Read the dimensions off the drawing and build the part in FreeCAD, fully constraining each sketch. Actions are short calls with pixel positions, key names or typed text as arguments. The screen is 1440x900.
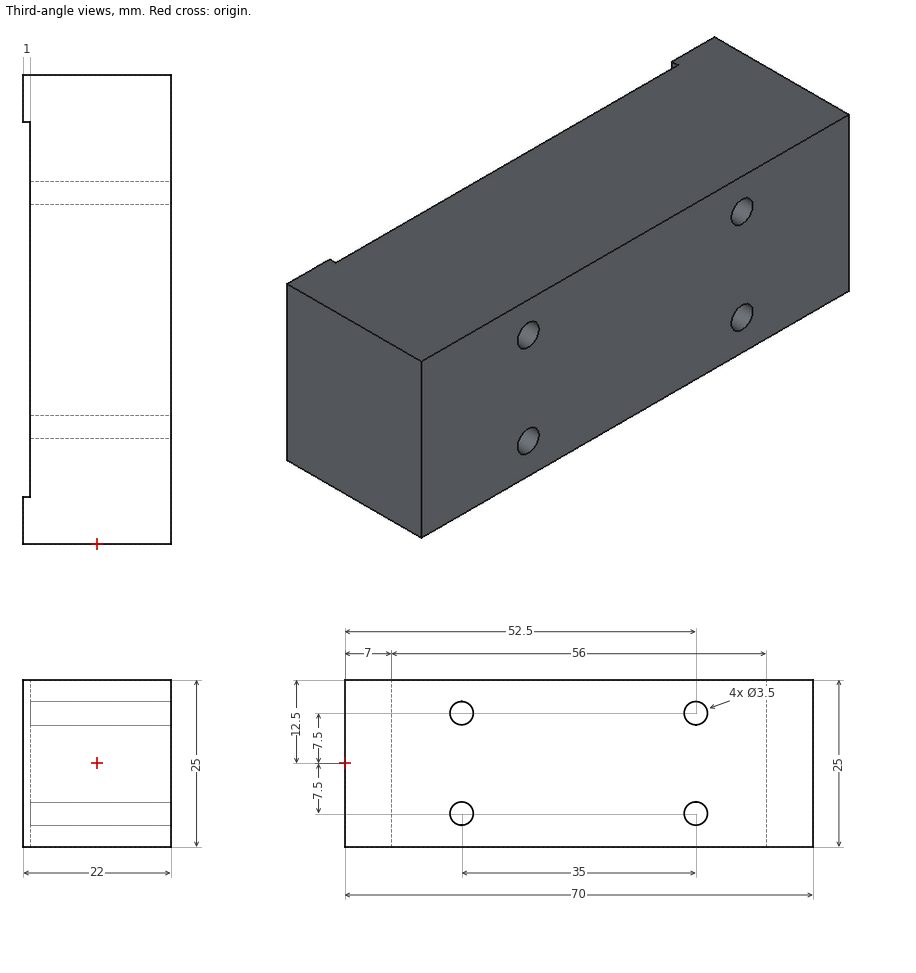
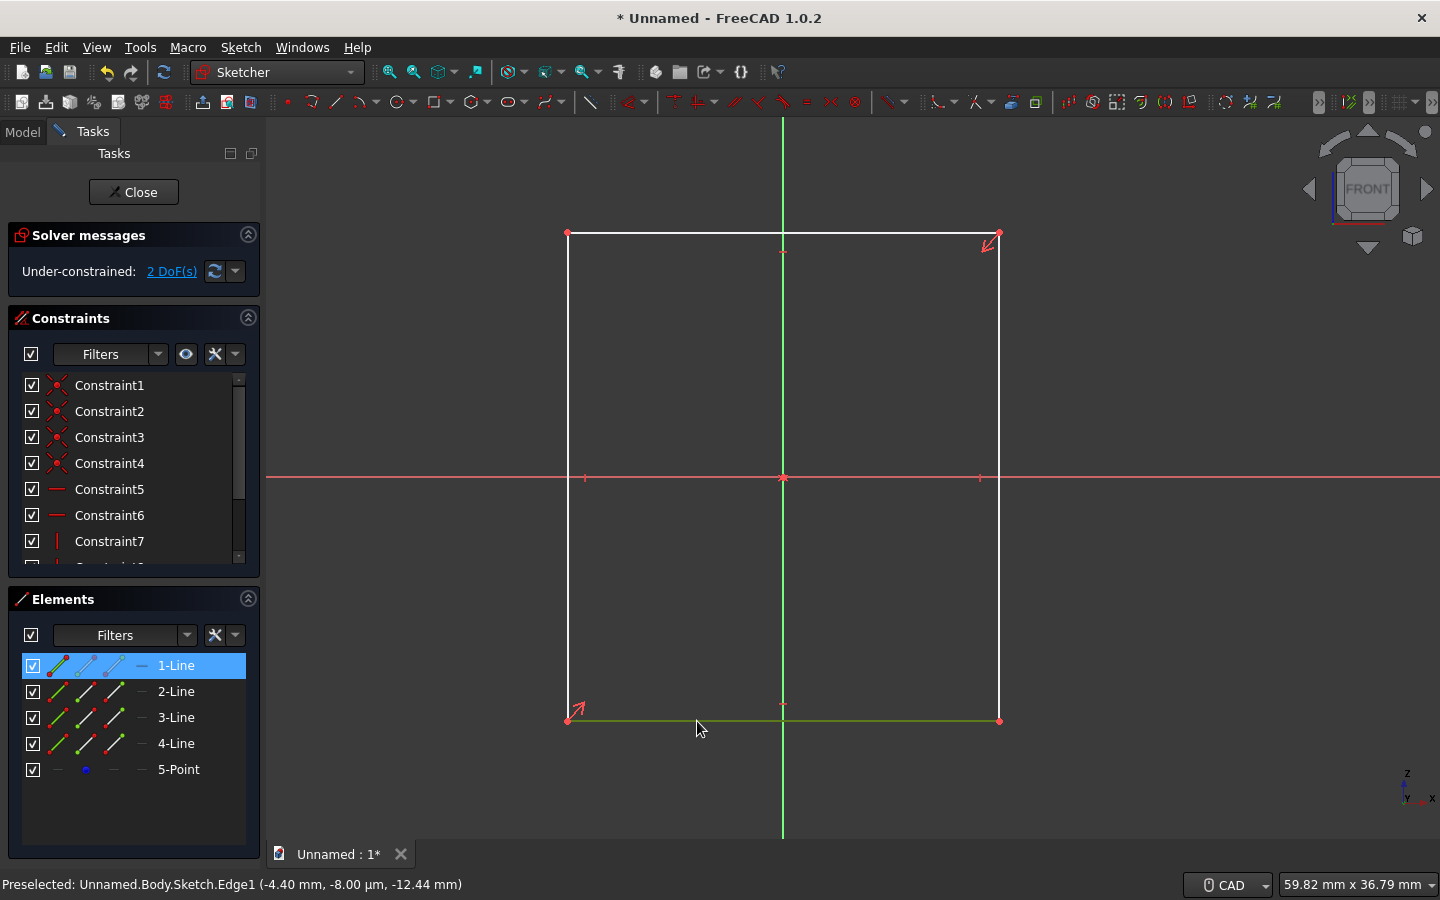
click(646, 102)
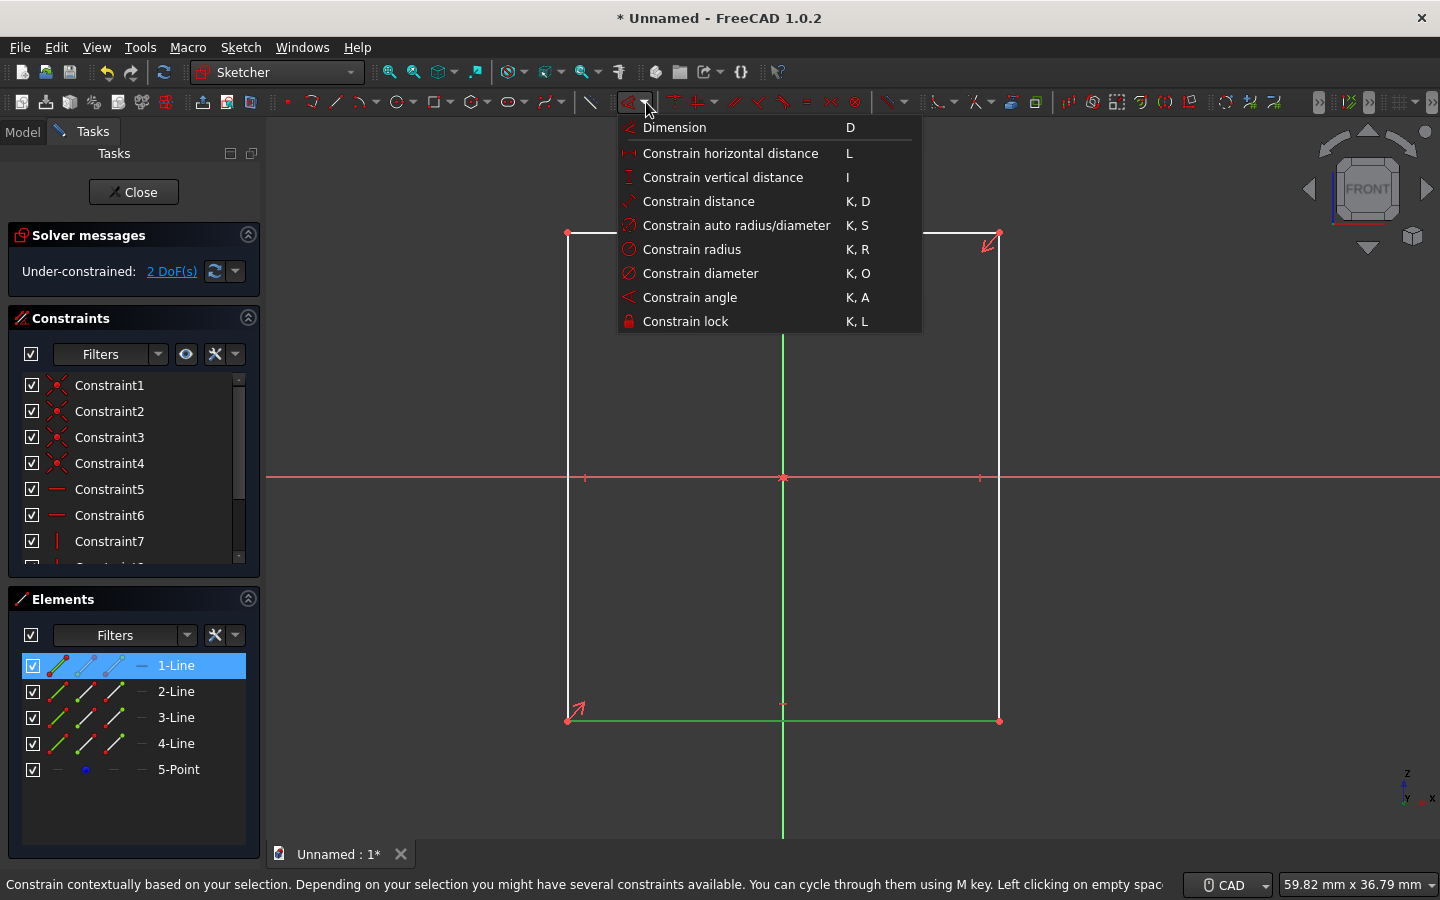
click(770, 153)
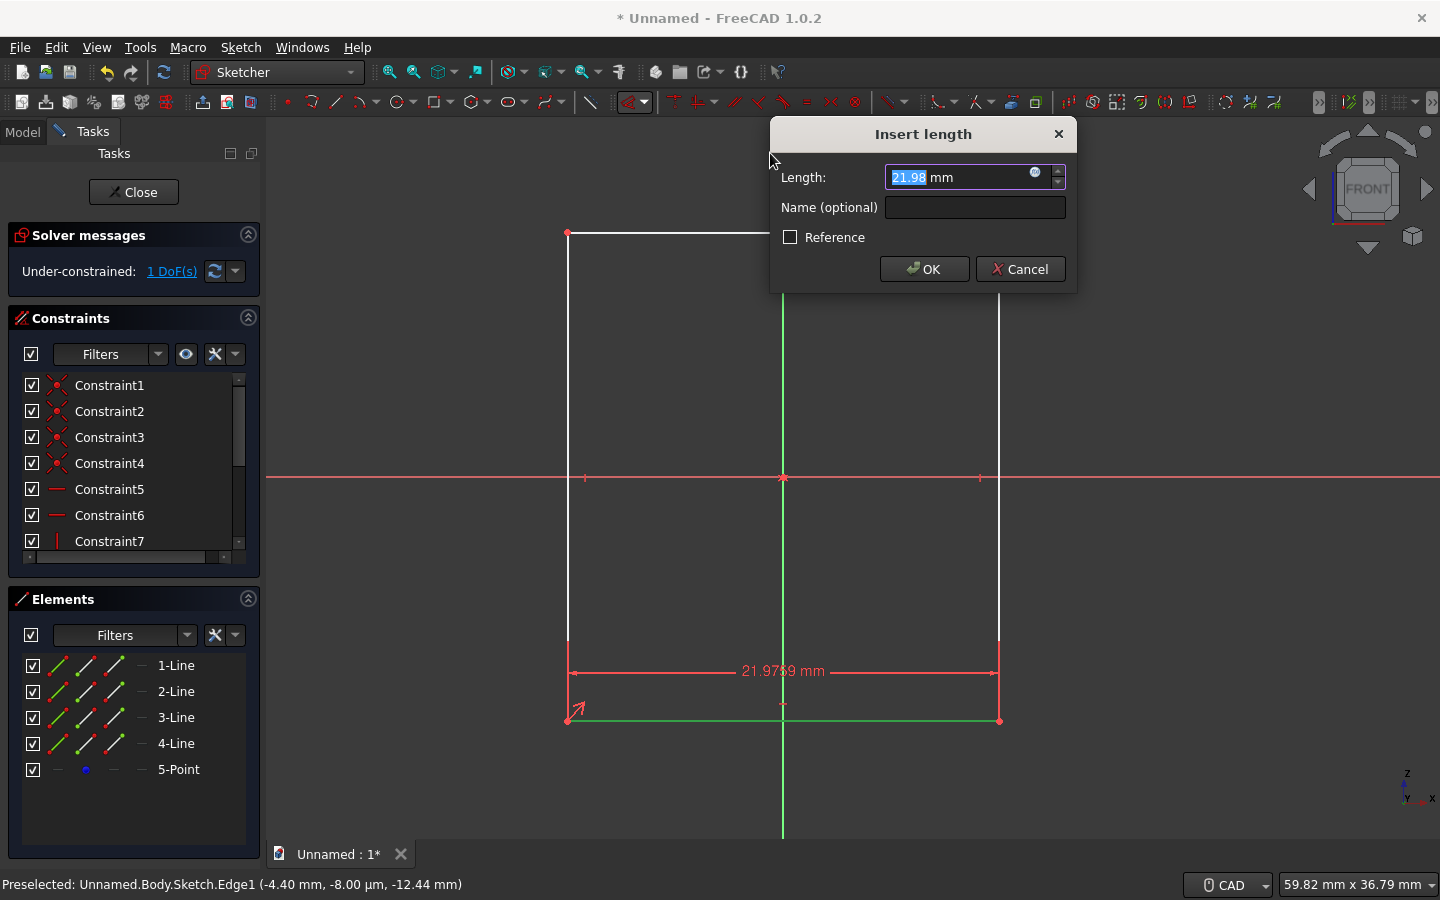
text(22)
key(Return)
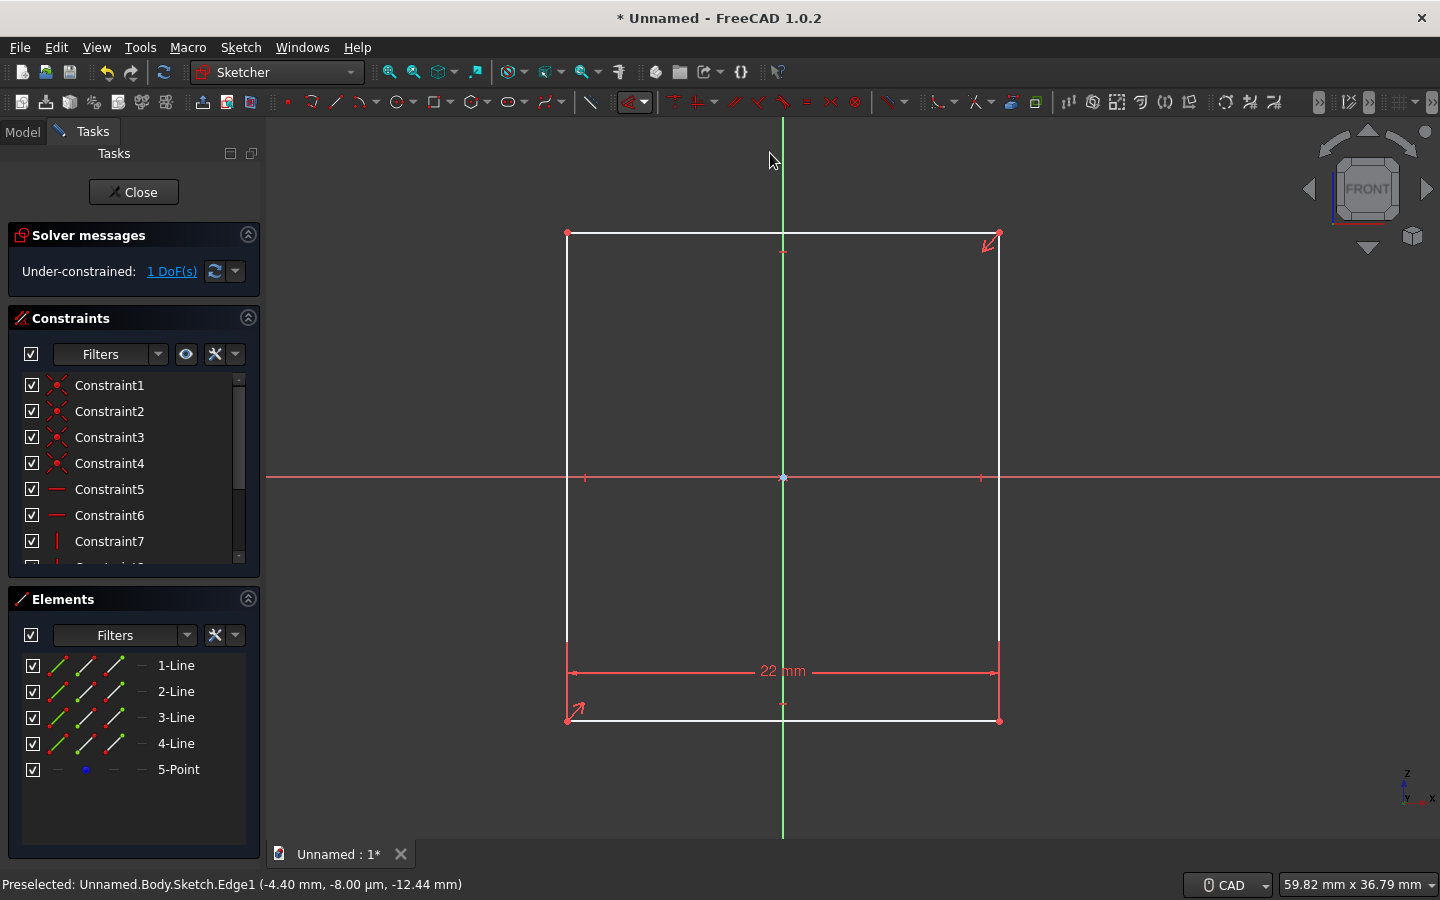
click(999, 575)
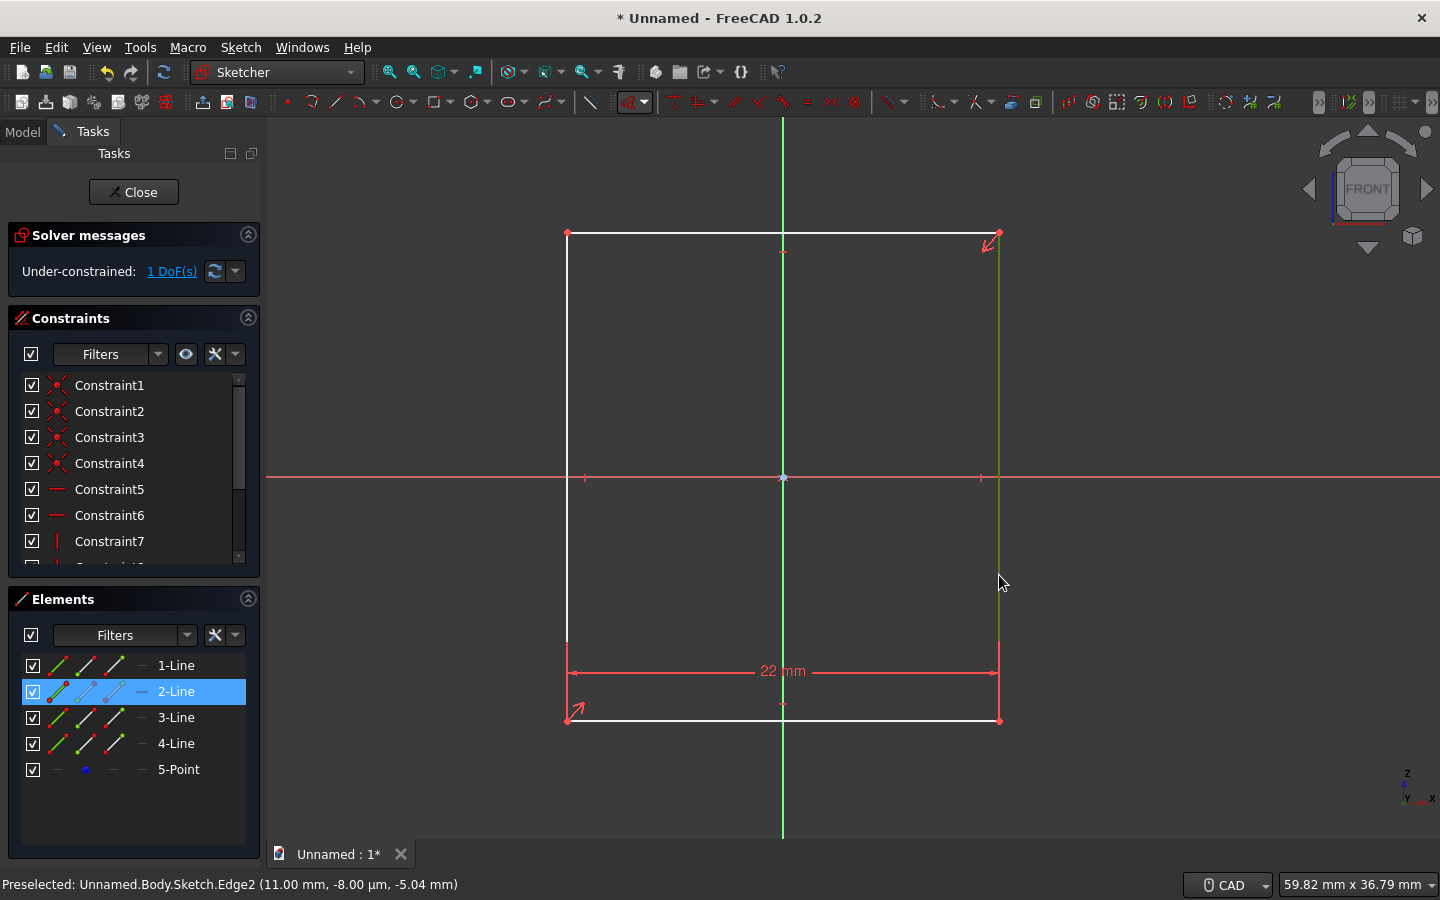
click(646, 102)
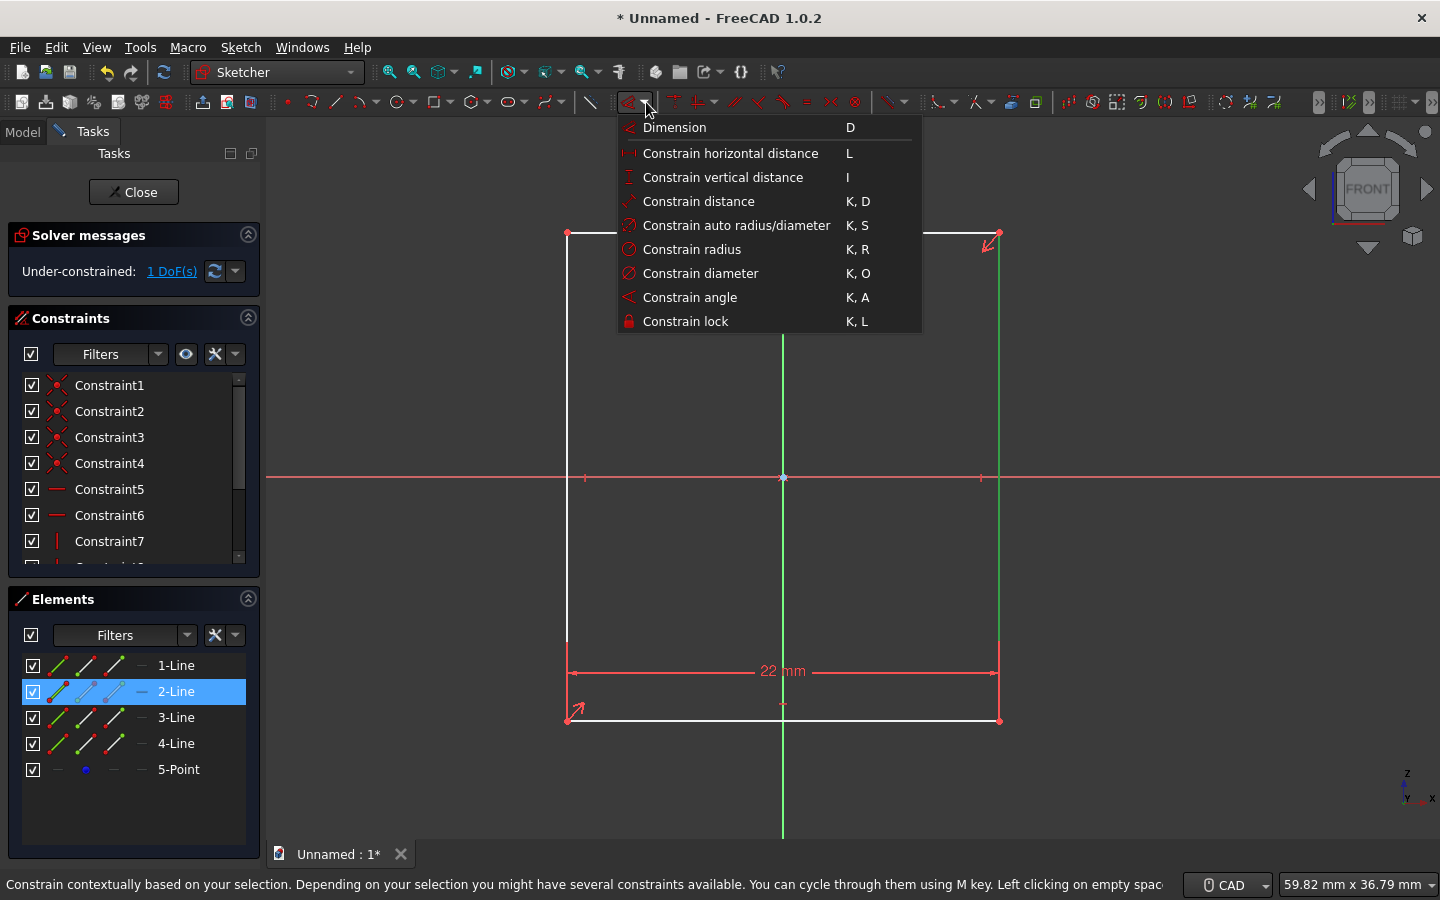
click(770, 177)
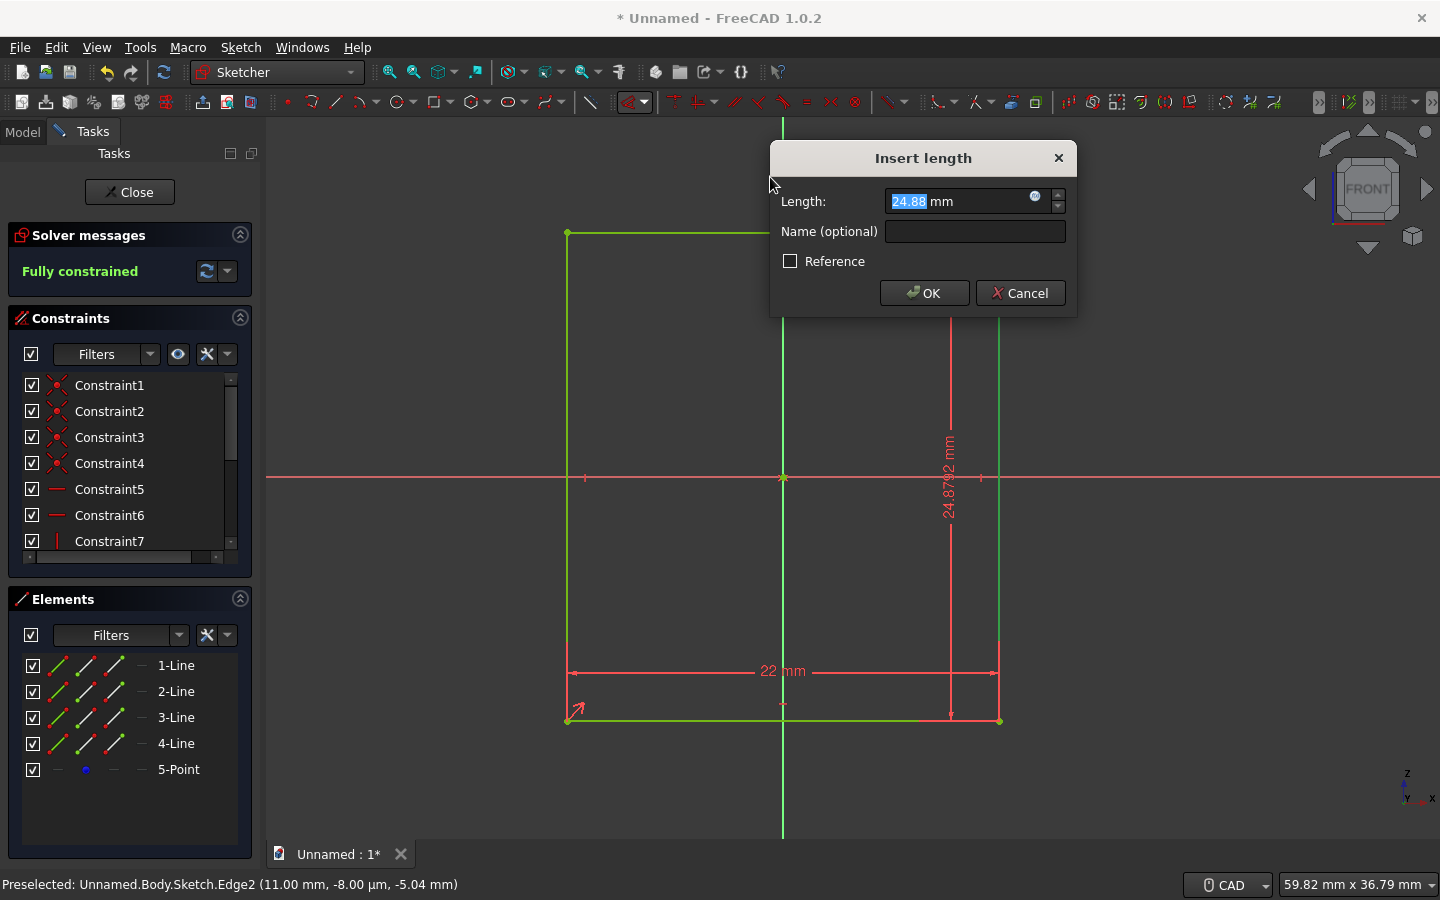
text(25)
key(Return)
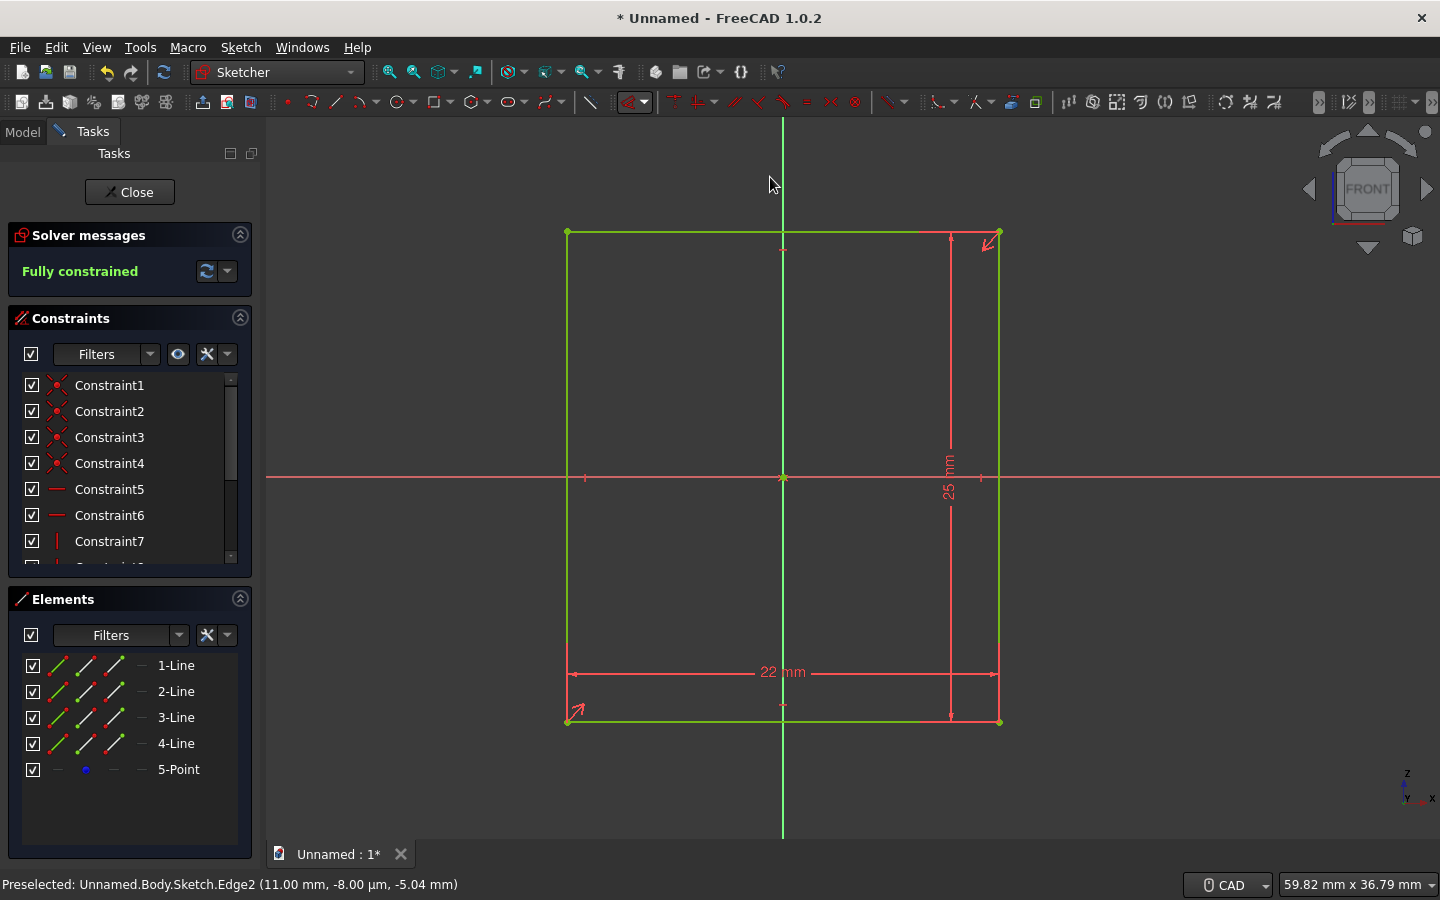
click(130, 192)